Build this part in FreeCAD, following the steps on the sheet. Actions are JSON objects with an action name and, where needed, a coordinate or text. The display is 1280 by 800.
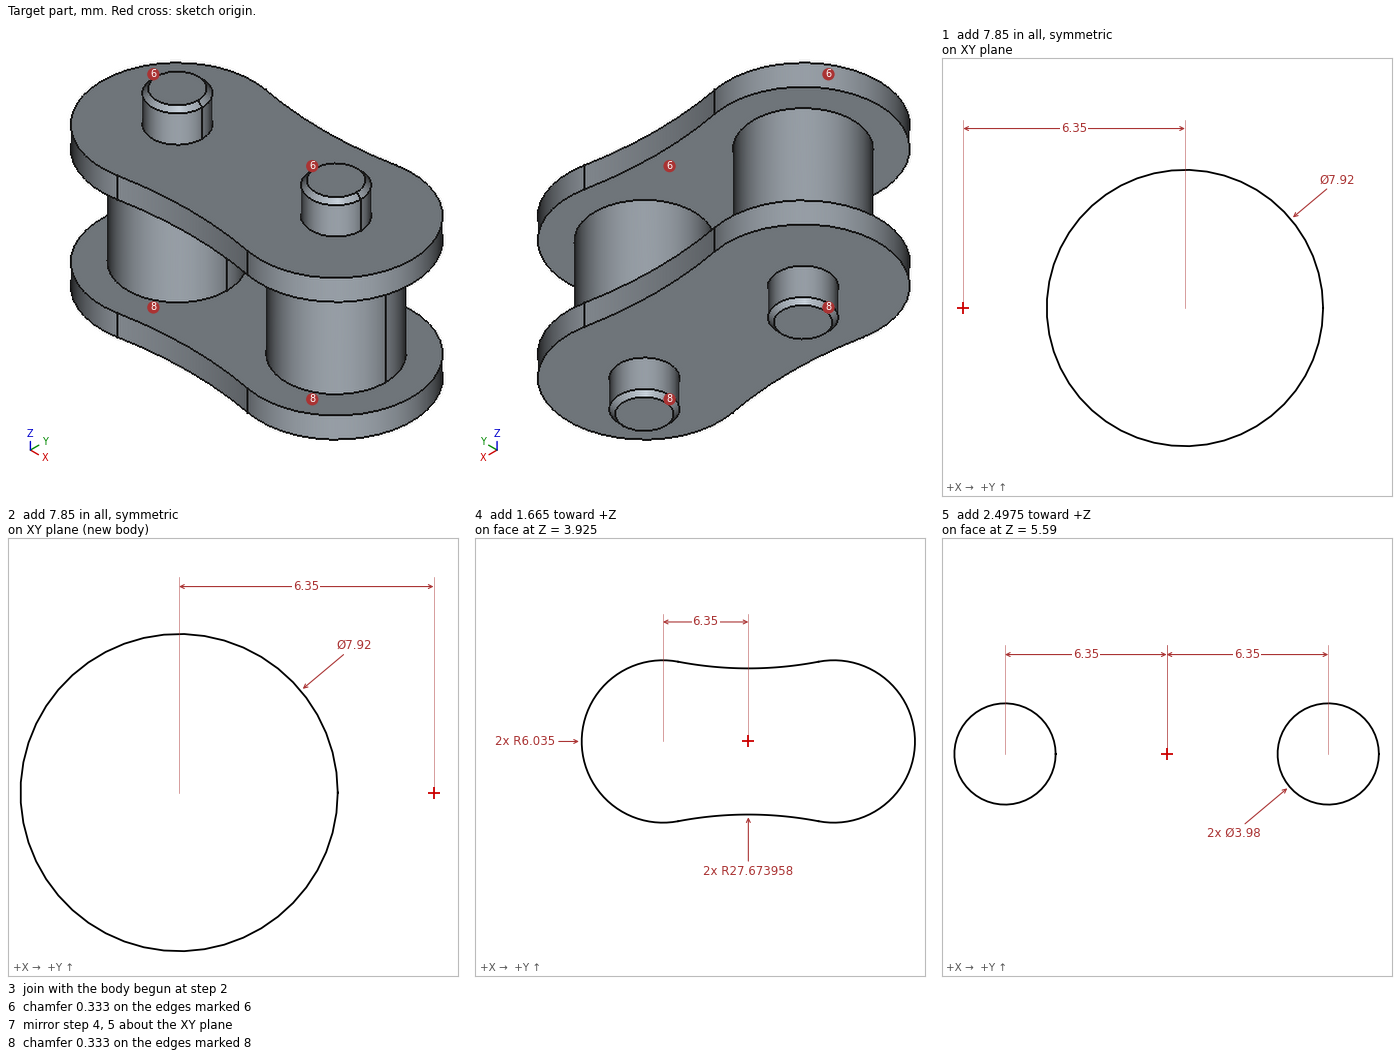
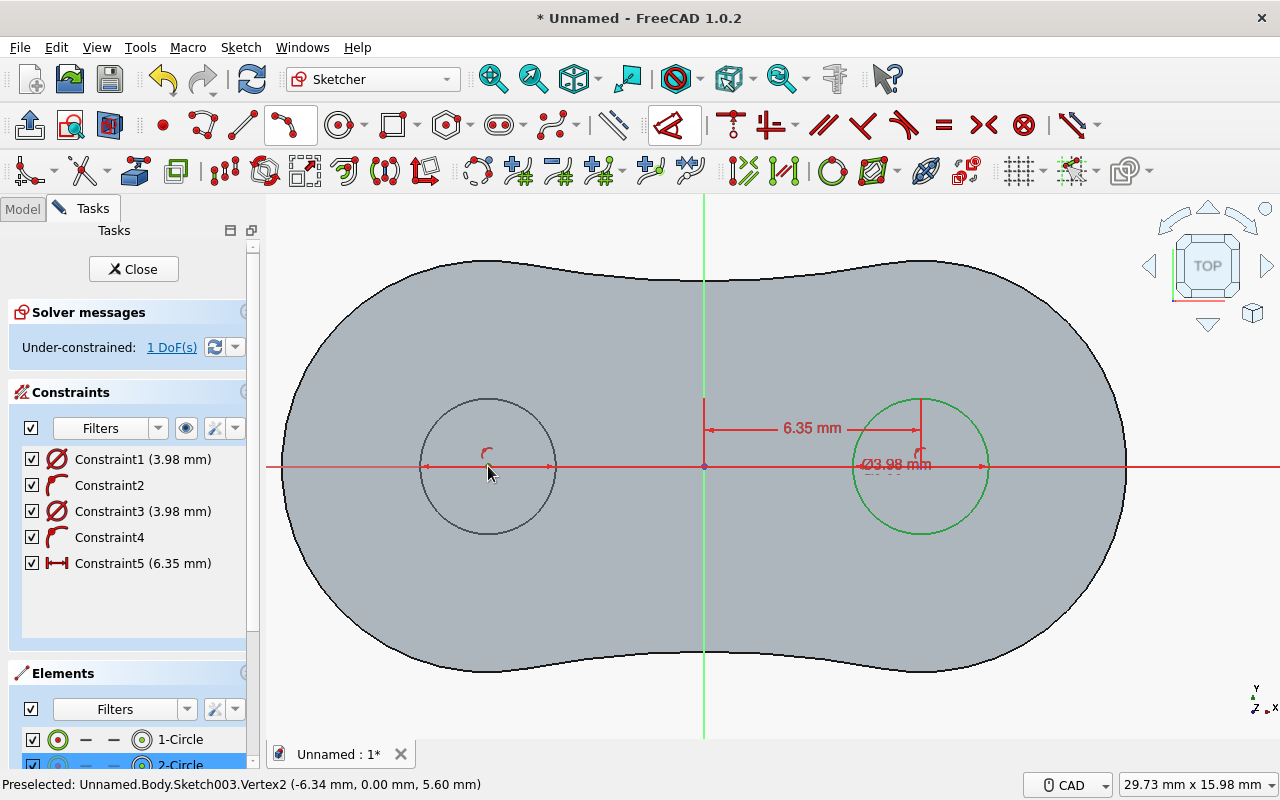
{"action": "left_click", "coordinate": [696, 126]}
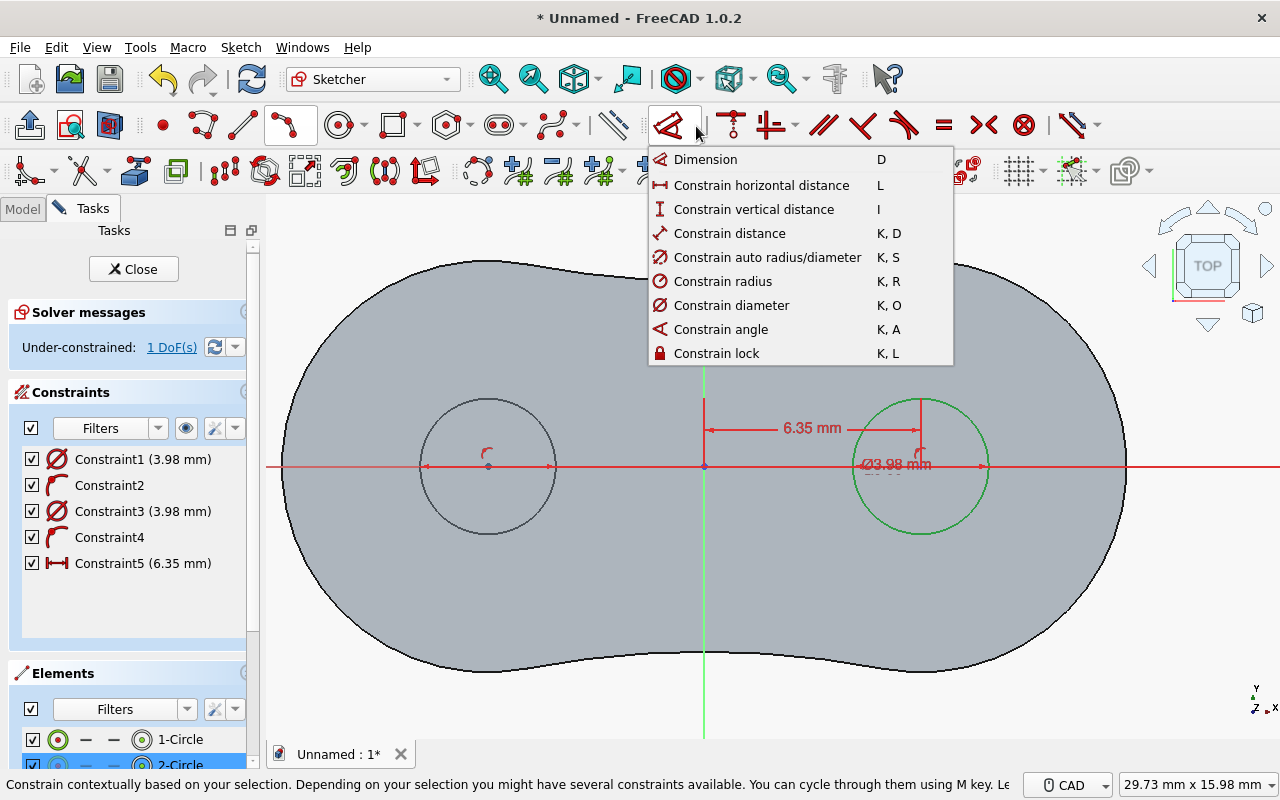
{"action": "left_click", "coordinate": [801, 185]}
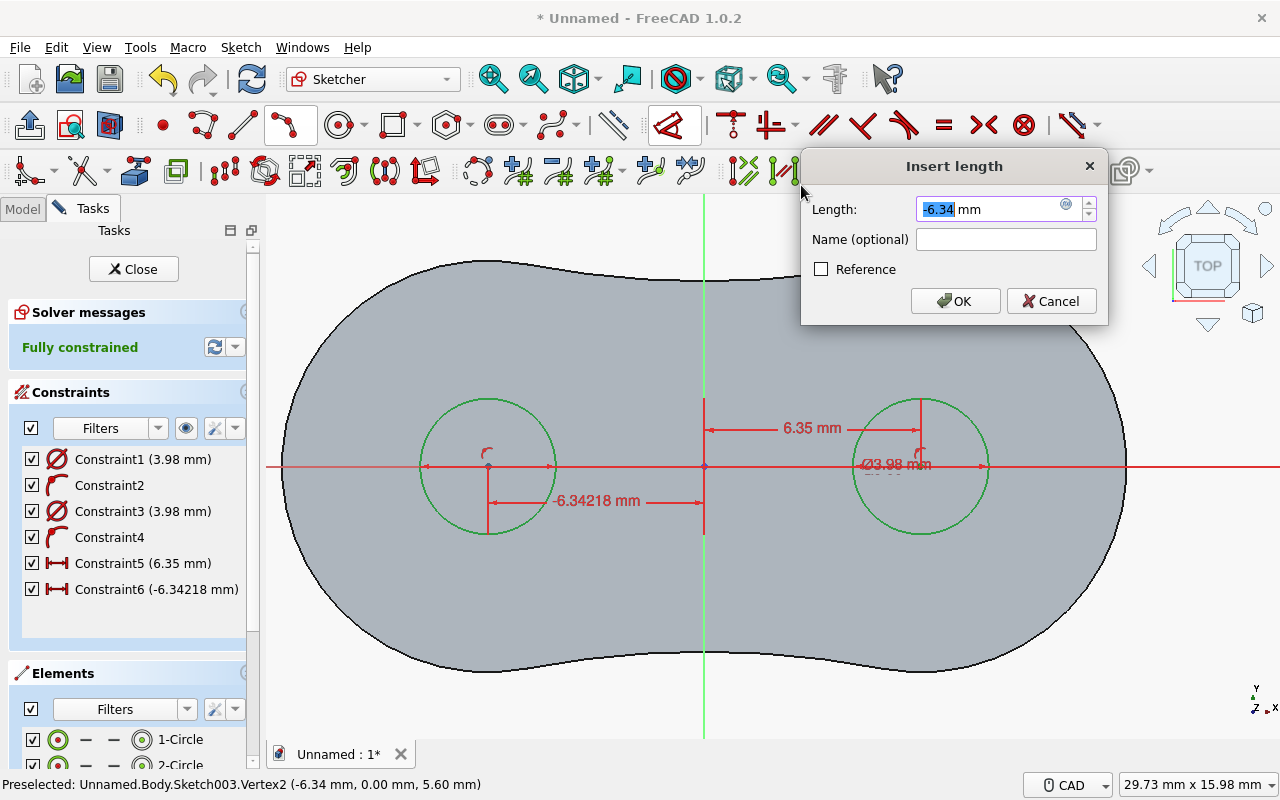
{"action": "type", "text": "-6.35"}
{"action": "key", "text": "Return"}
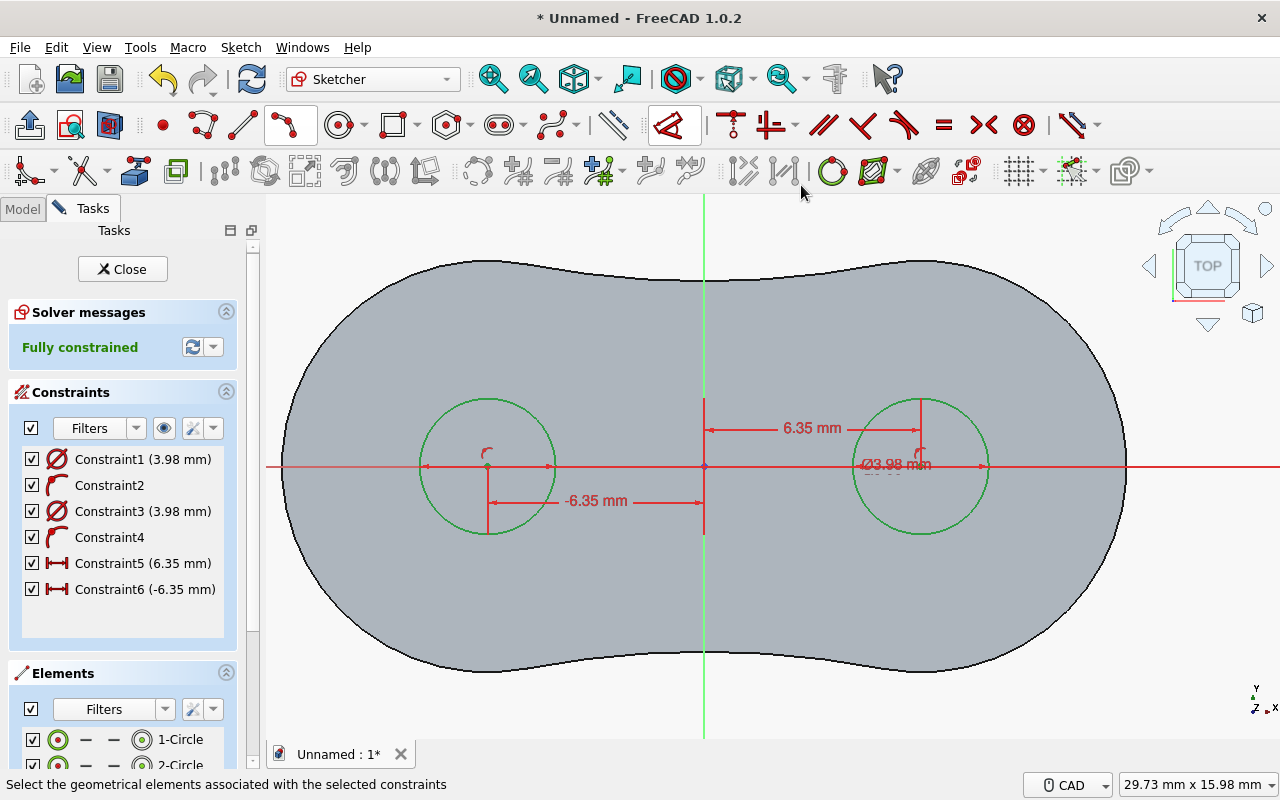
{"action": "left_click", "coordinate": [123, 269]}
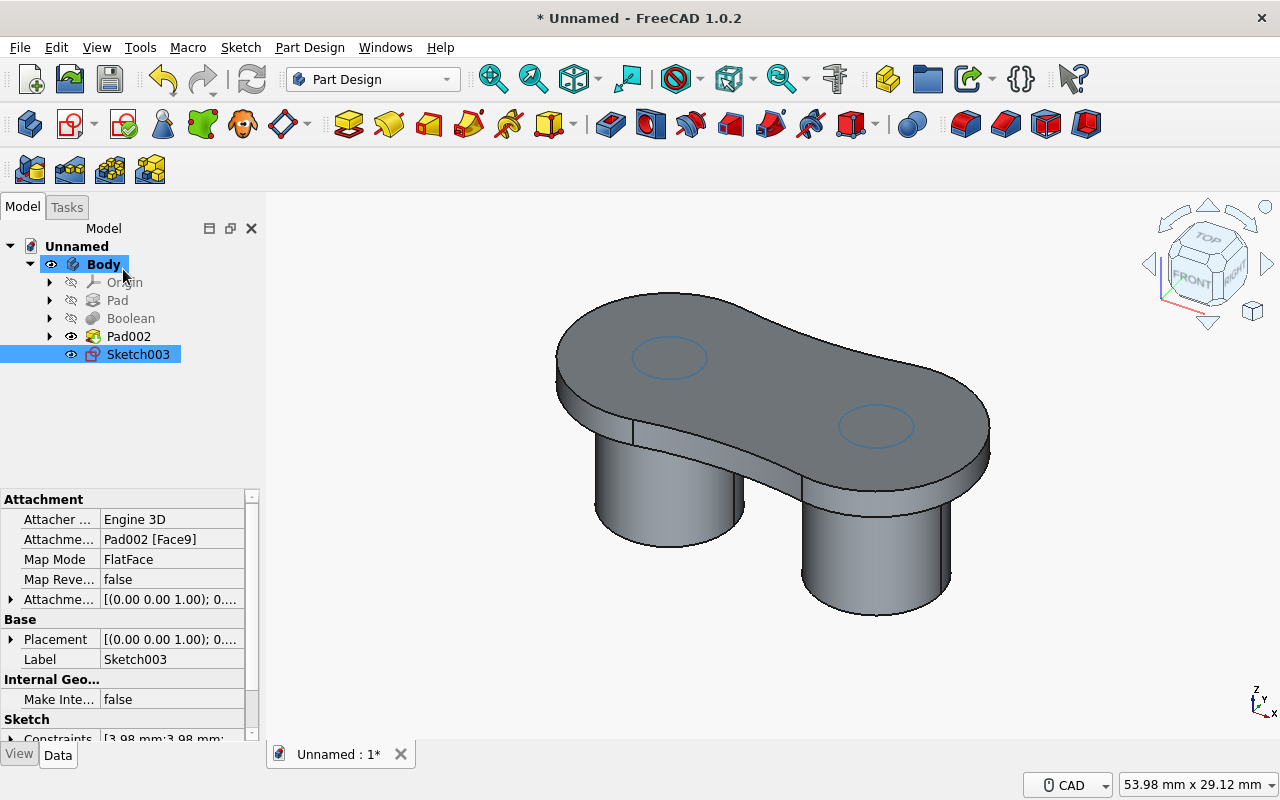
{"action": "left_click", "coordinate": [350, 124]}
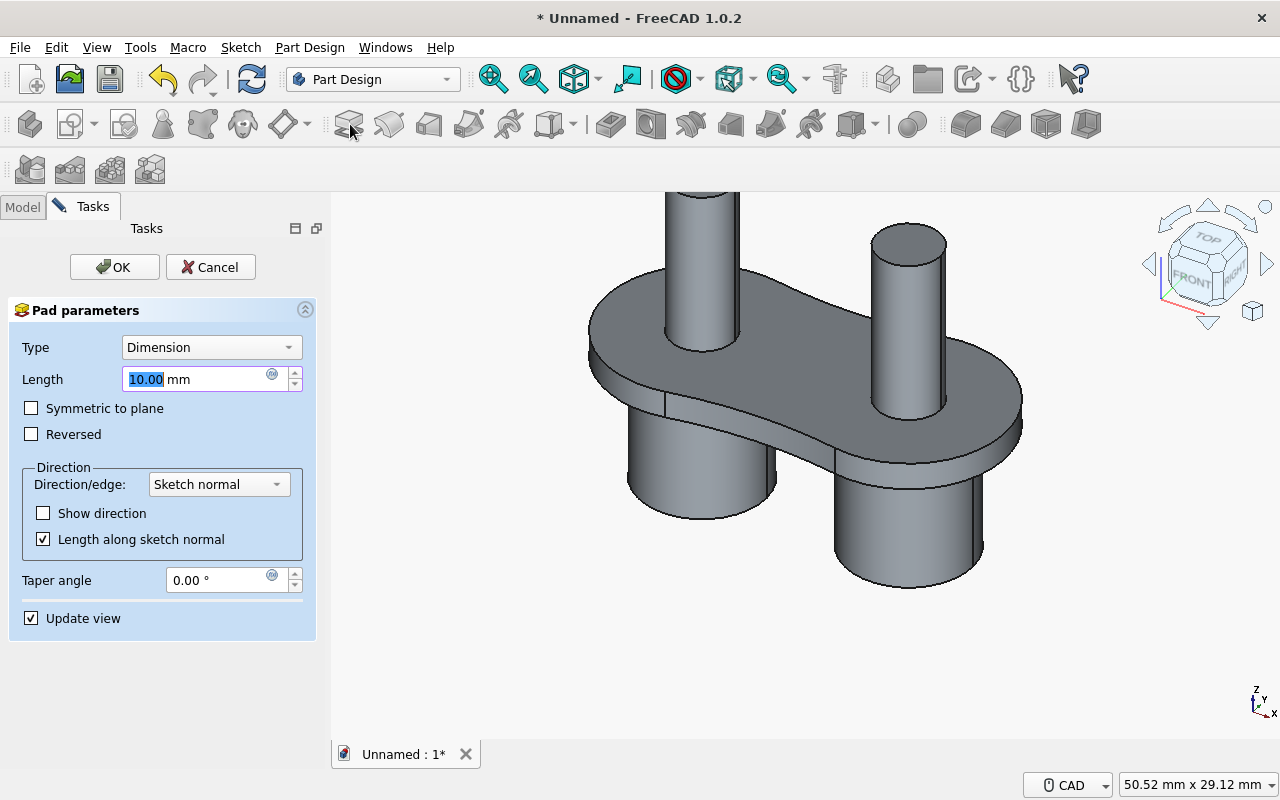
{"action": "type", "text": "2.4975"}
{"action": "key", "text": "Tab"}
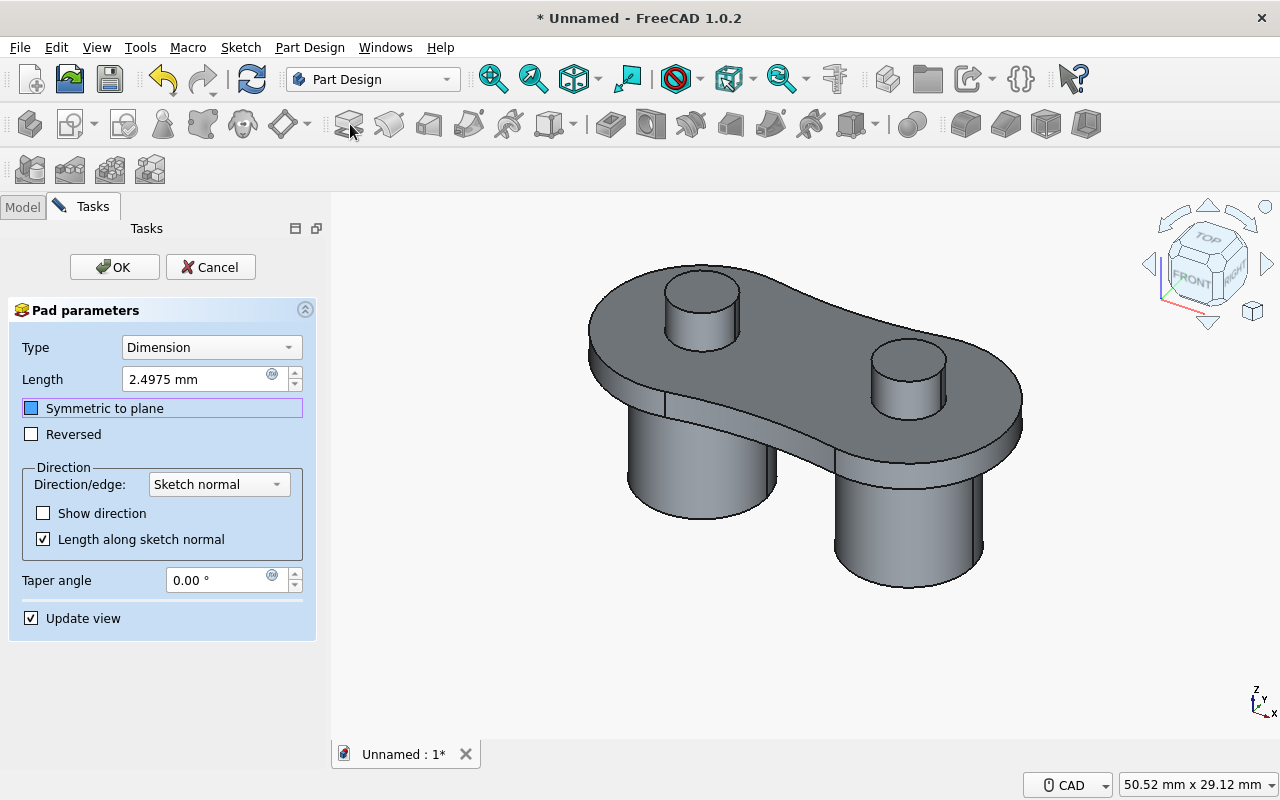
{"action": "left_click", "coordinate": [115, 267]}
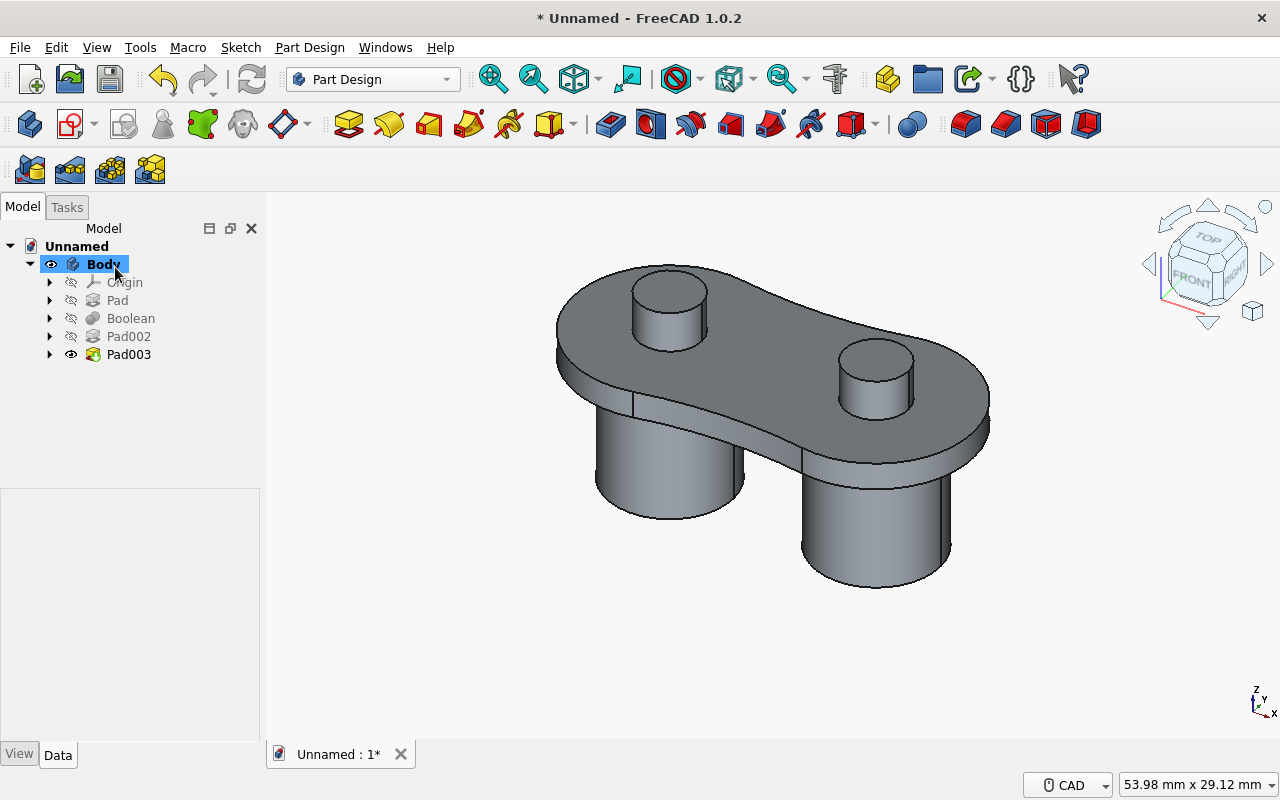
{"action": "left_click", "coordinate": [839, 361]}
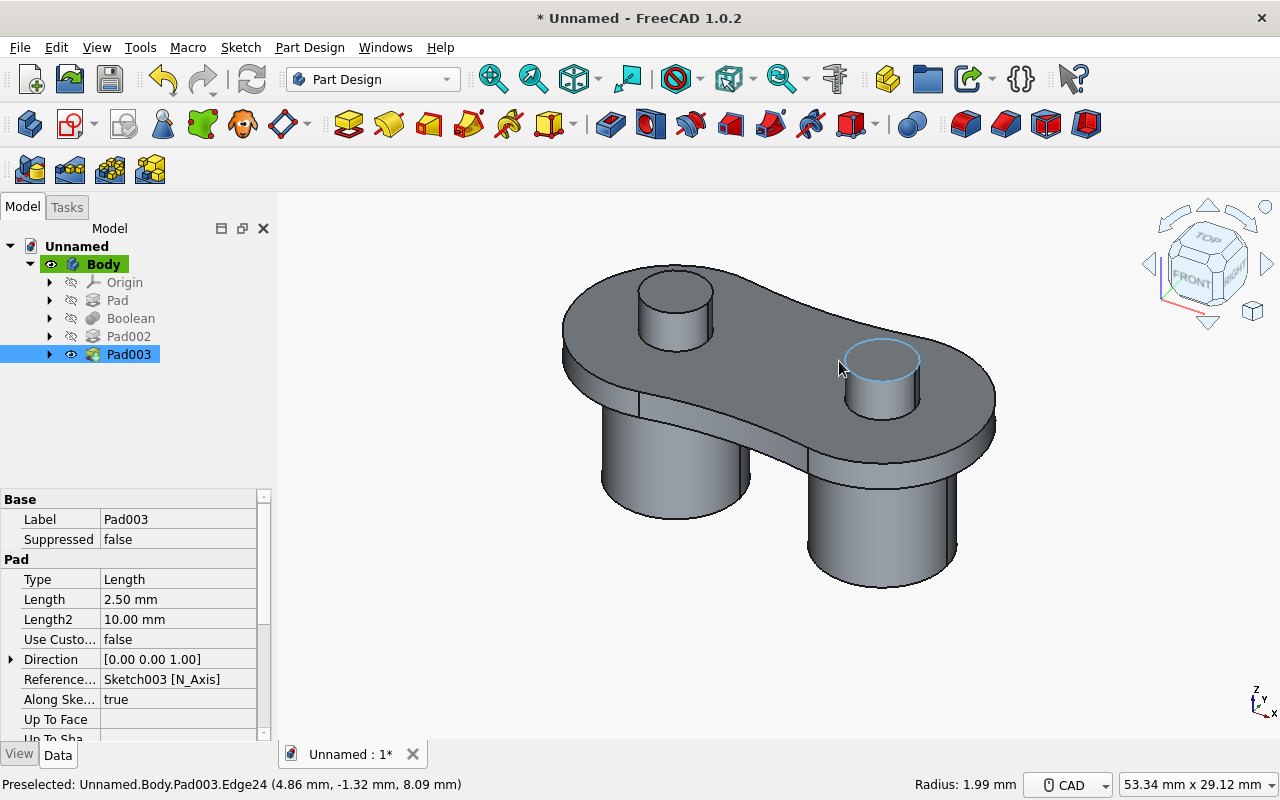
{"action": "left_click", "coordinate": [639, 293], "text": "ctrl"}